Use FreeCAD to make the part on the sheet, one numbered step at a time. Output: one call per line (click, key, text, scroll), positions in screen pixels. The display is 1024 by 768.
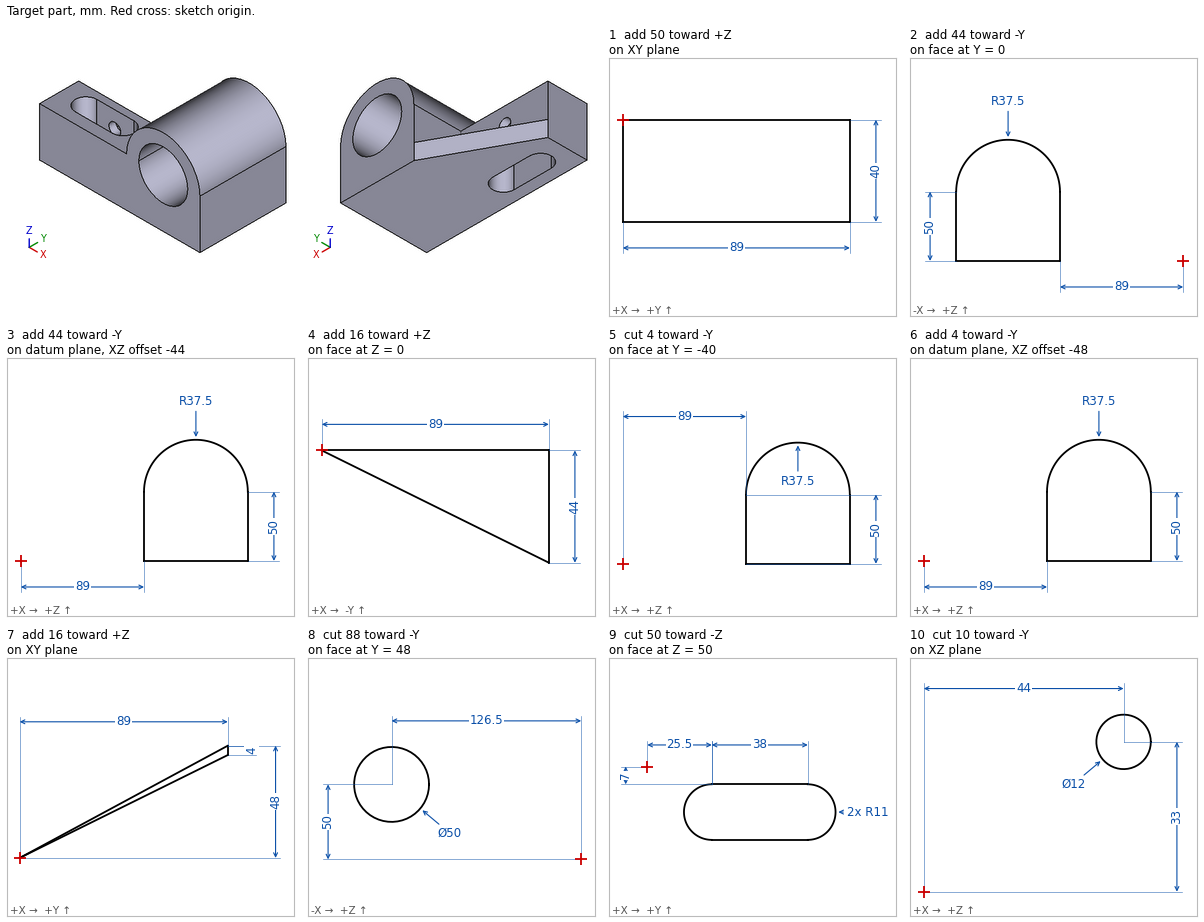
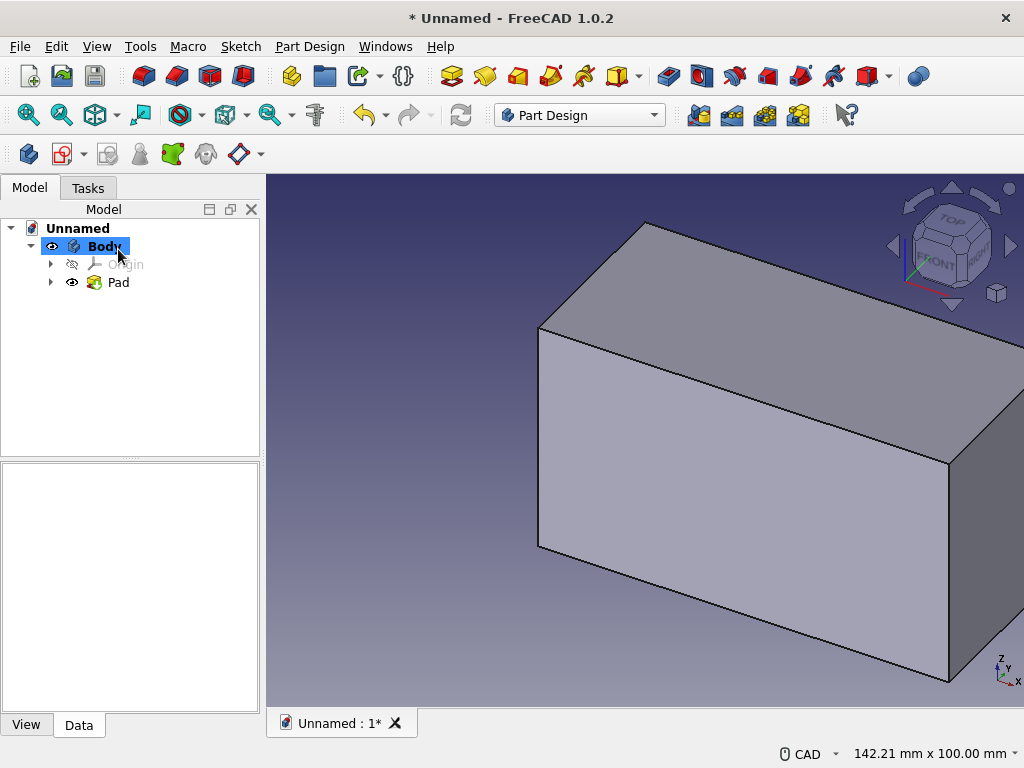
click(29, 116)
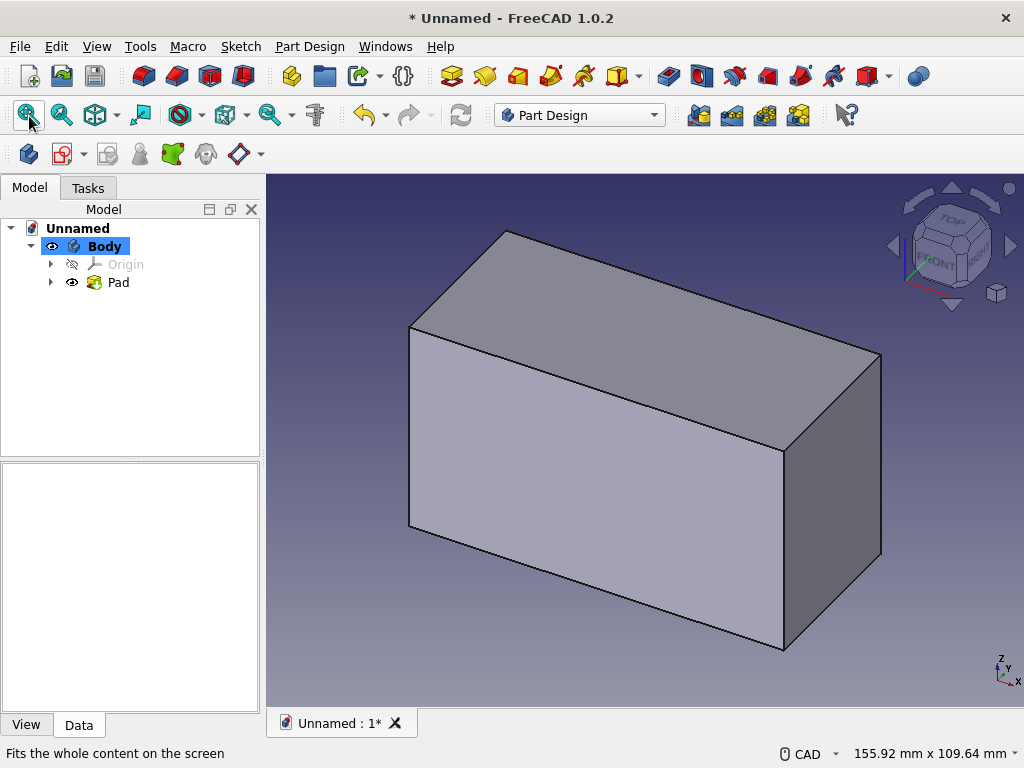
key(4)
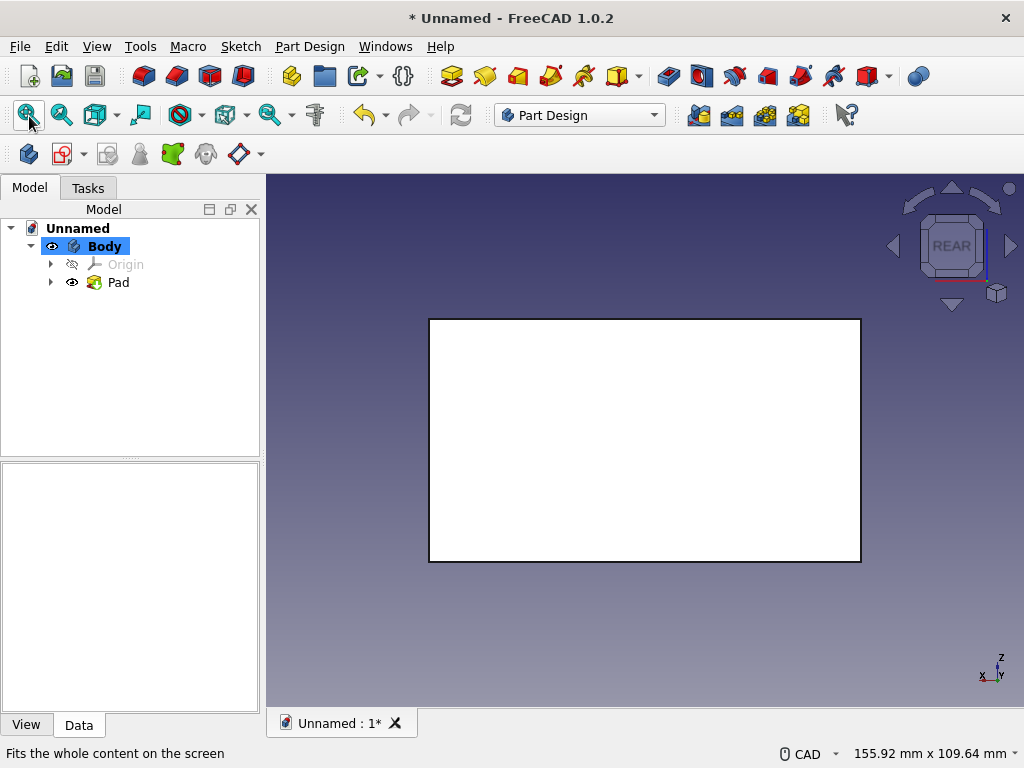
click(583, 439)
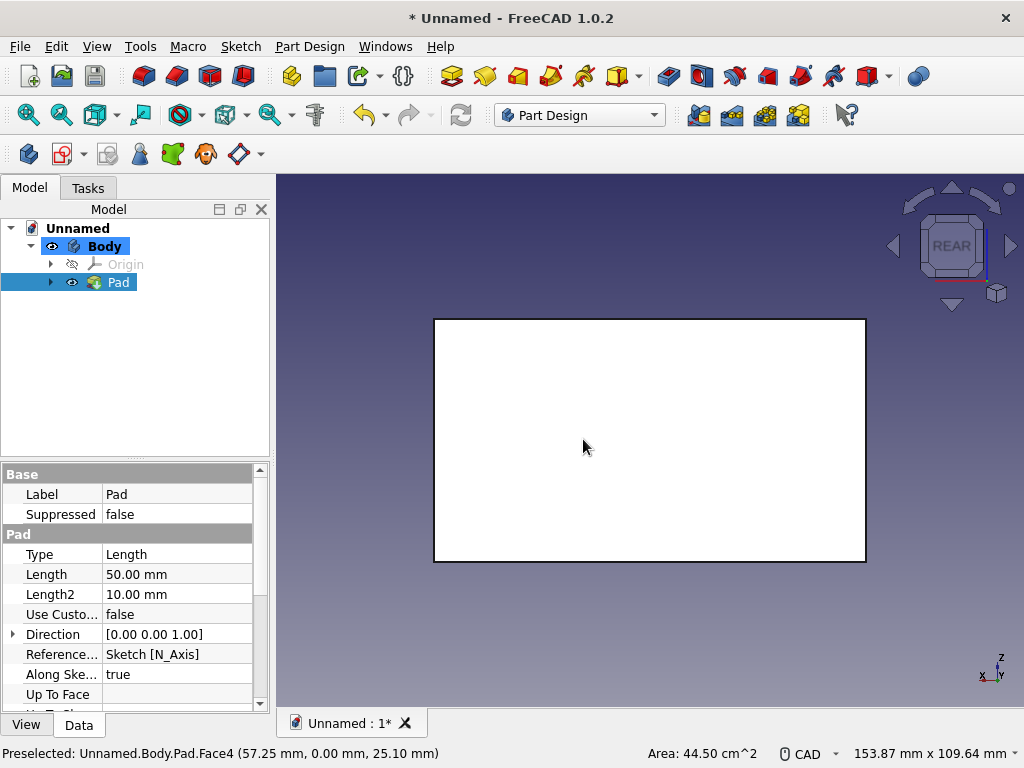
click(62, 154)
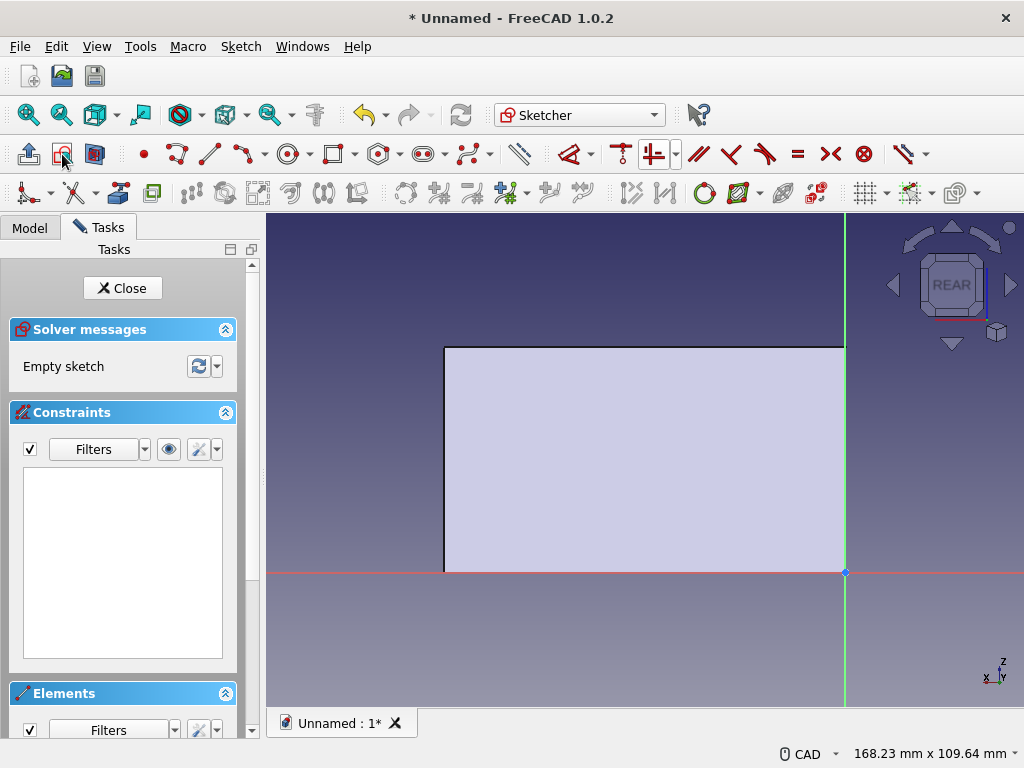
scroll(699, 563, down, 3)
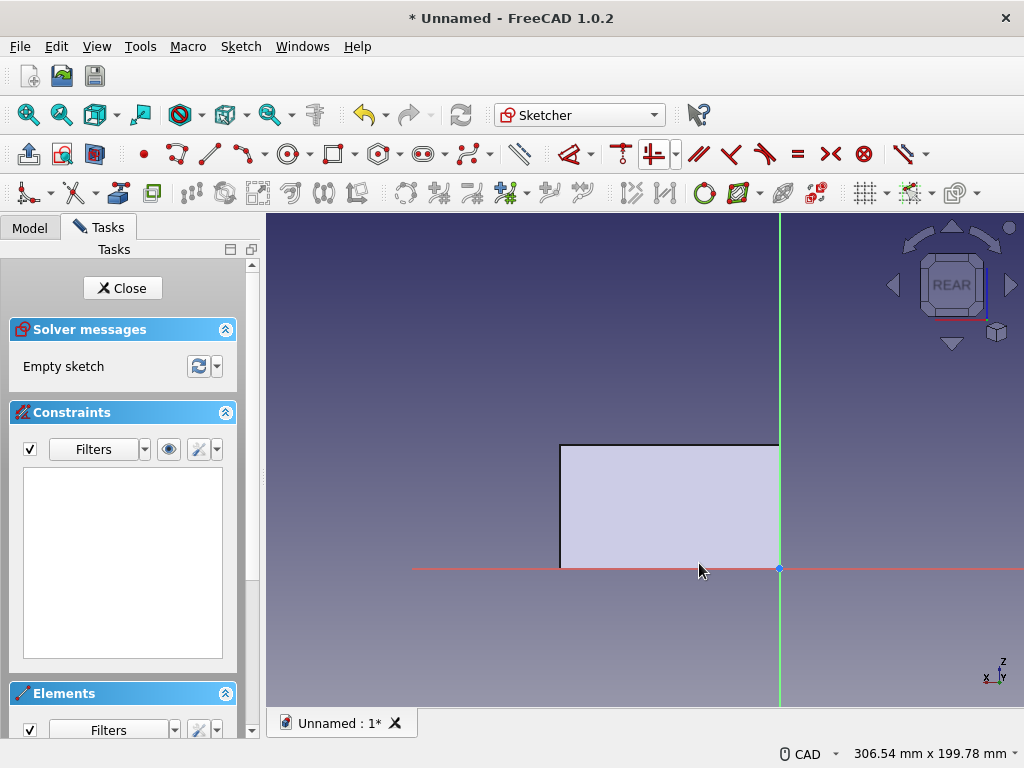
click(177, 154)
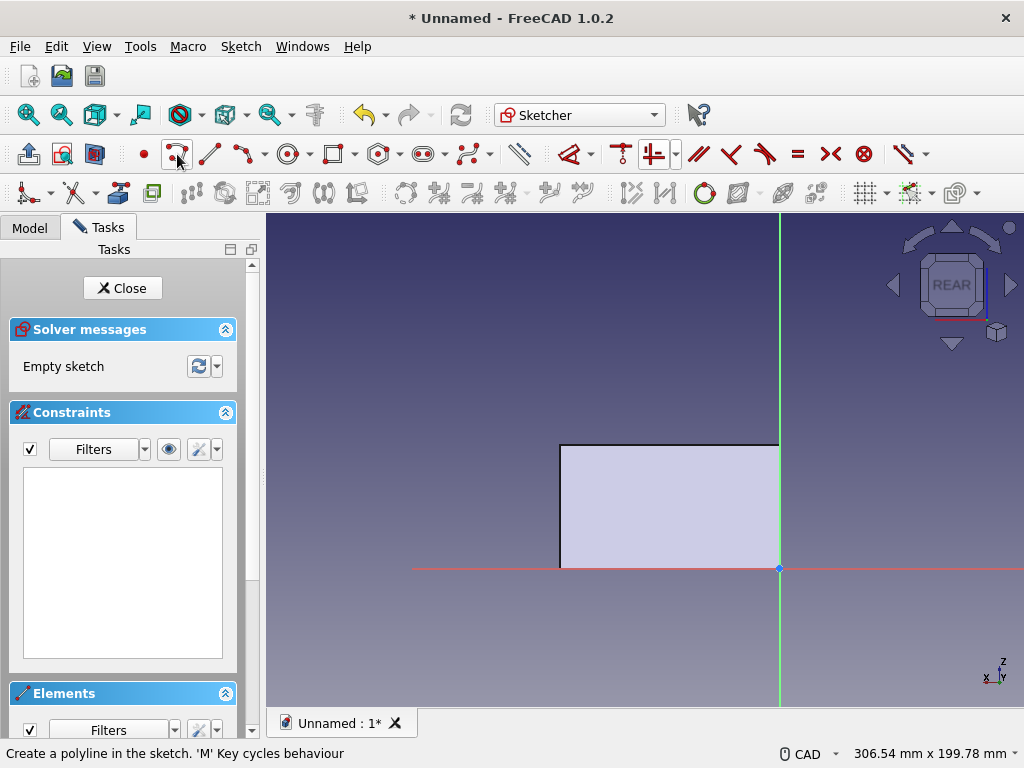
click(374, 445)
click(374, 569)
click(560, 560)
click(560, 445)
right_click(560, 445)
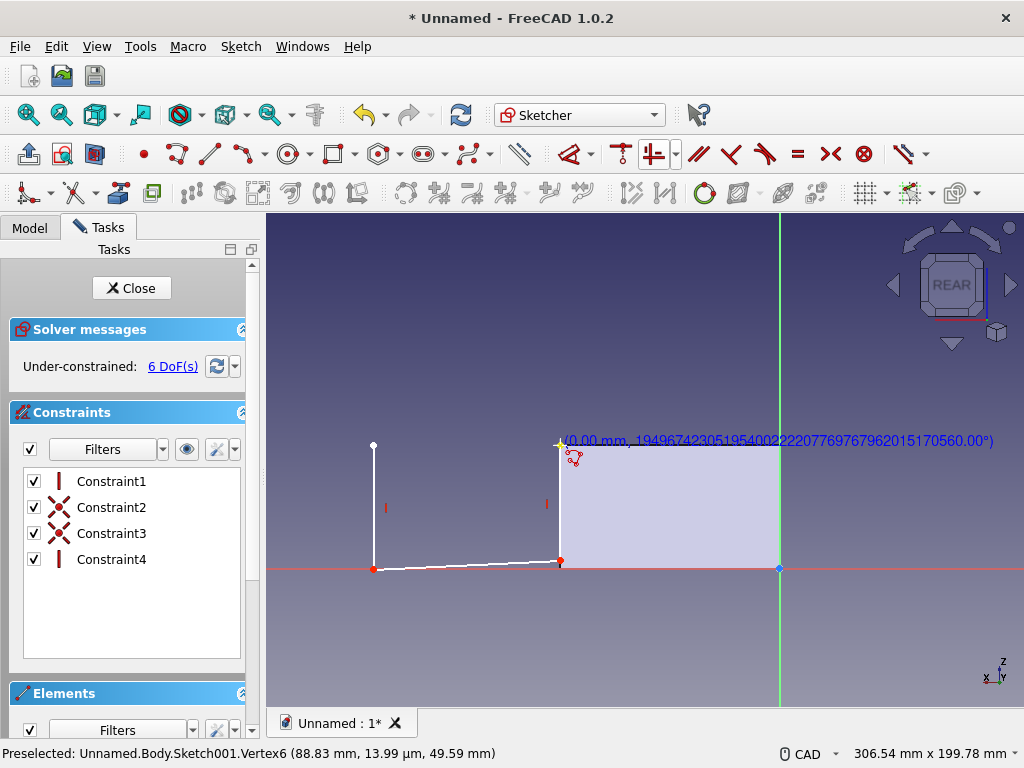
click(242, 154)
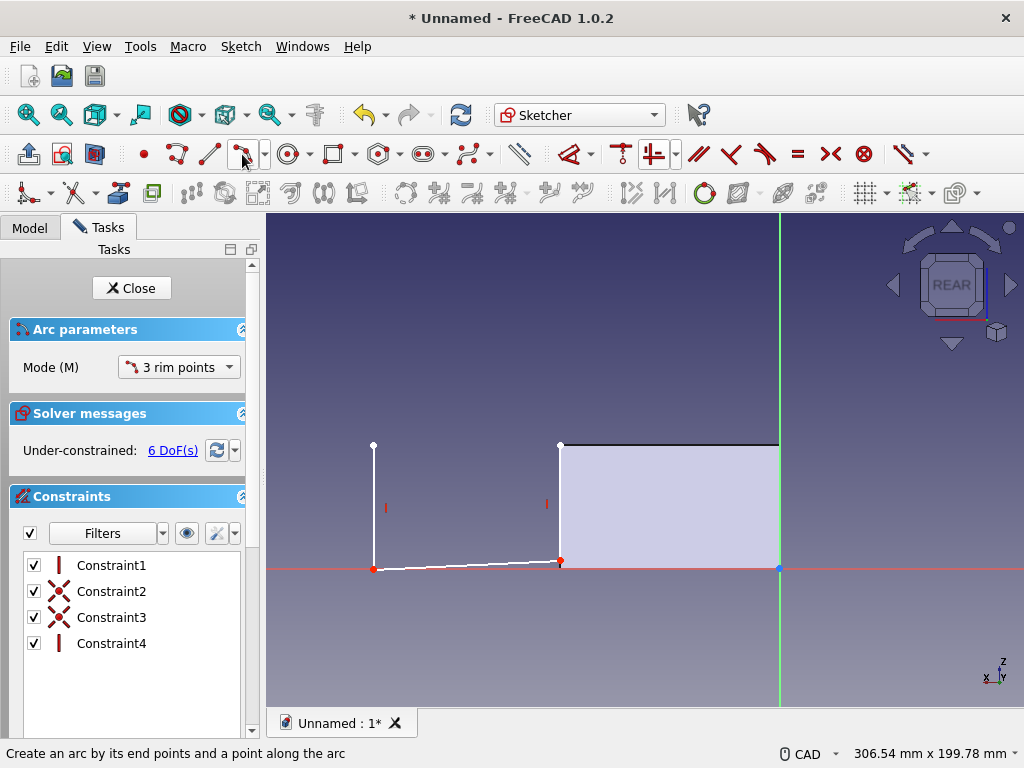
click(560, 446)
click(374, 446)
click(467, 352)
key(Escape)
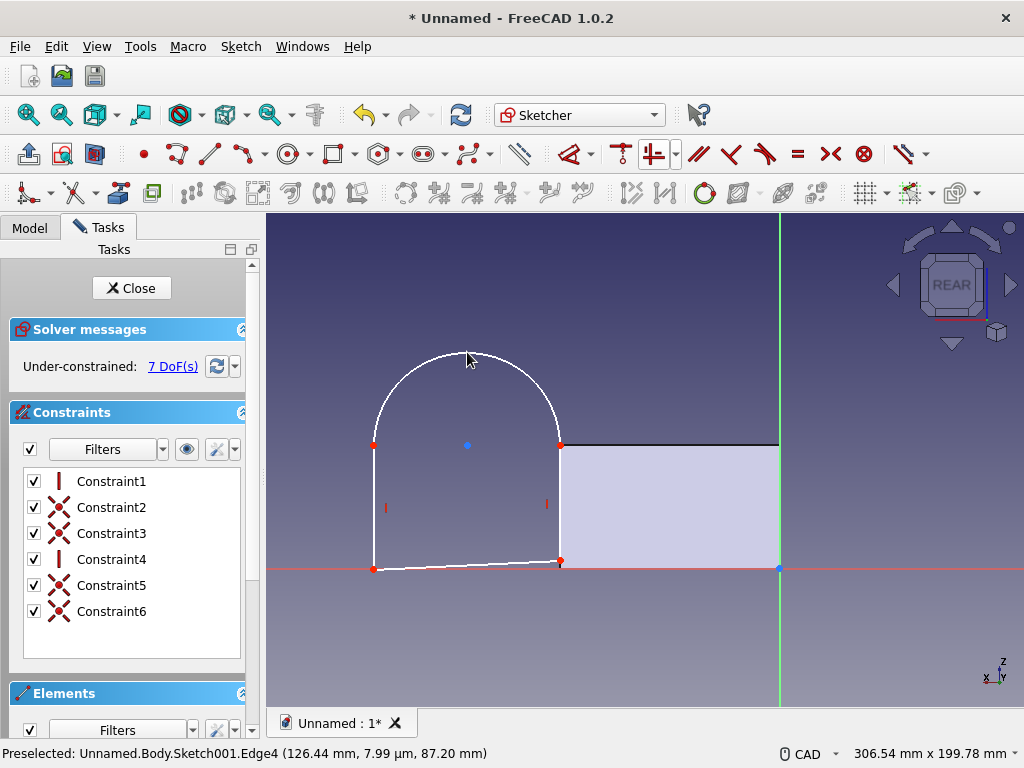
click(374, 483)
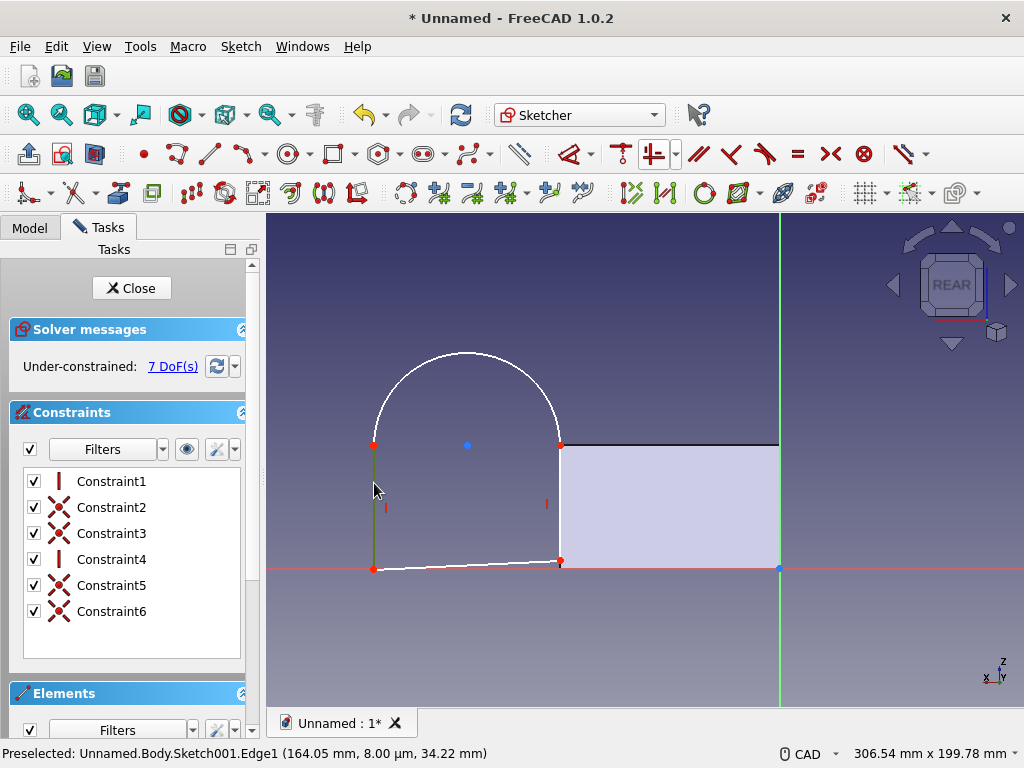
click(522, 371)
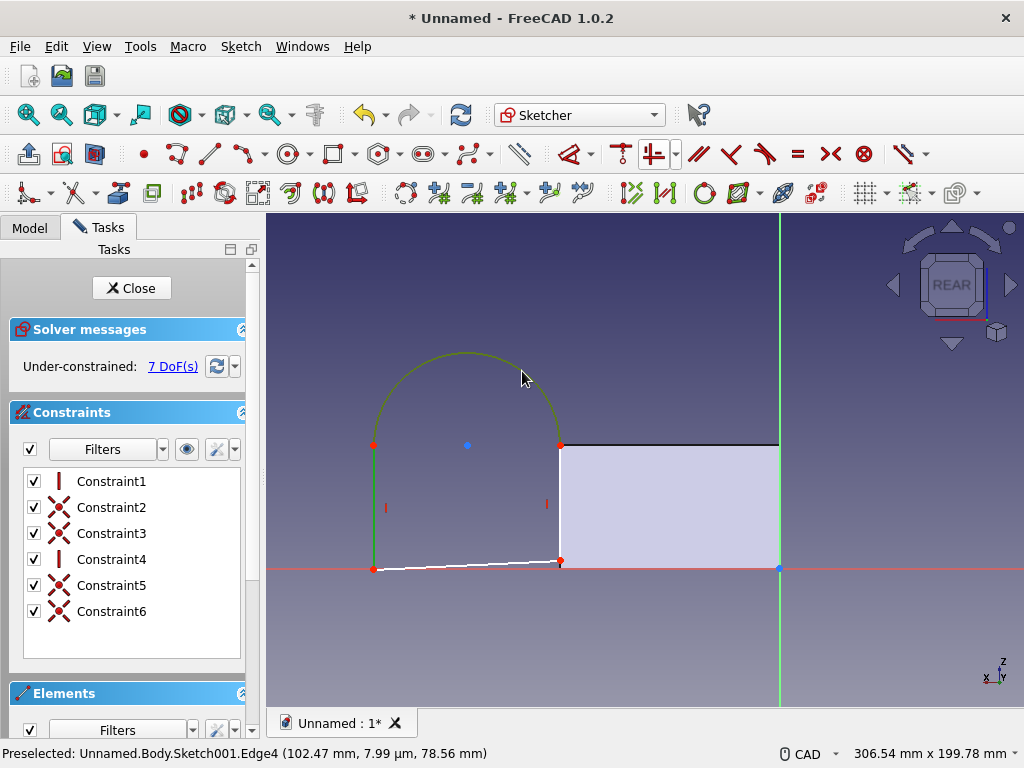
click(765, 154)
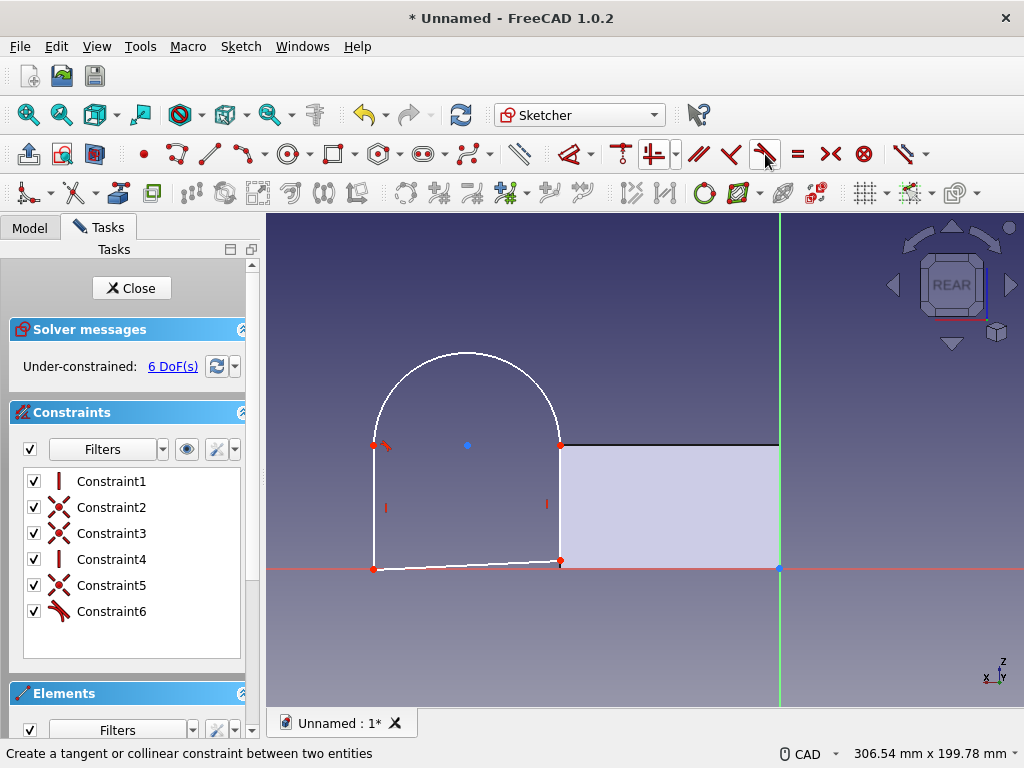
click(560, 527)